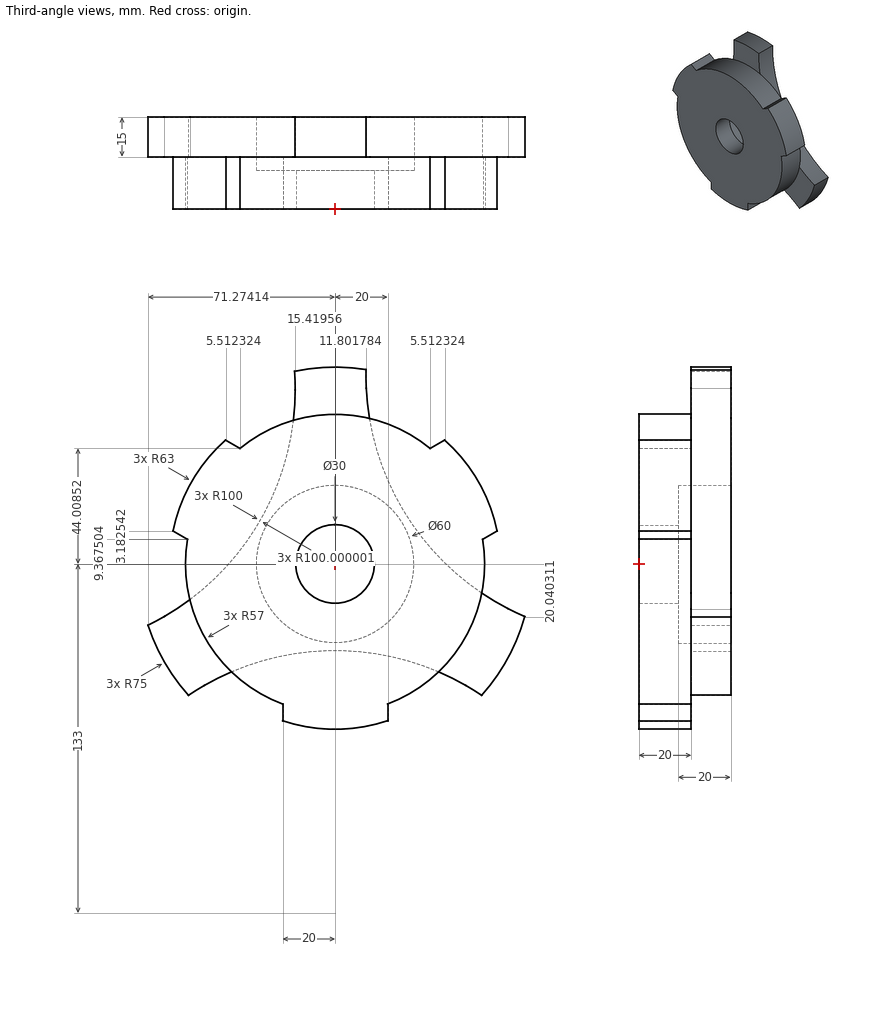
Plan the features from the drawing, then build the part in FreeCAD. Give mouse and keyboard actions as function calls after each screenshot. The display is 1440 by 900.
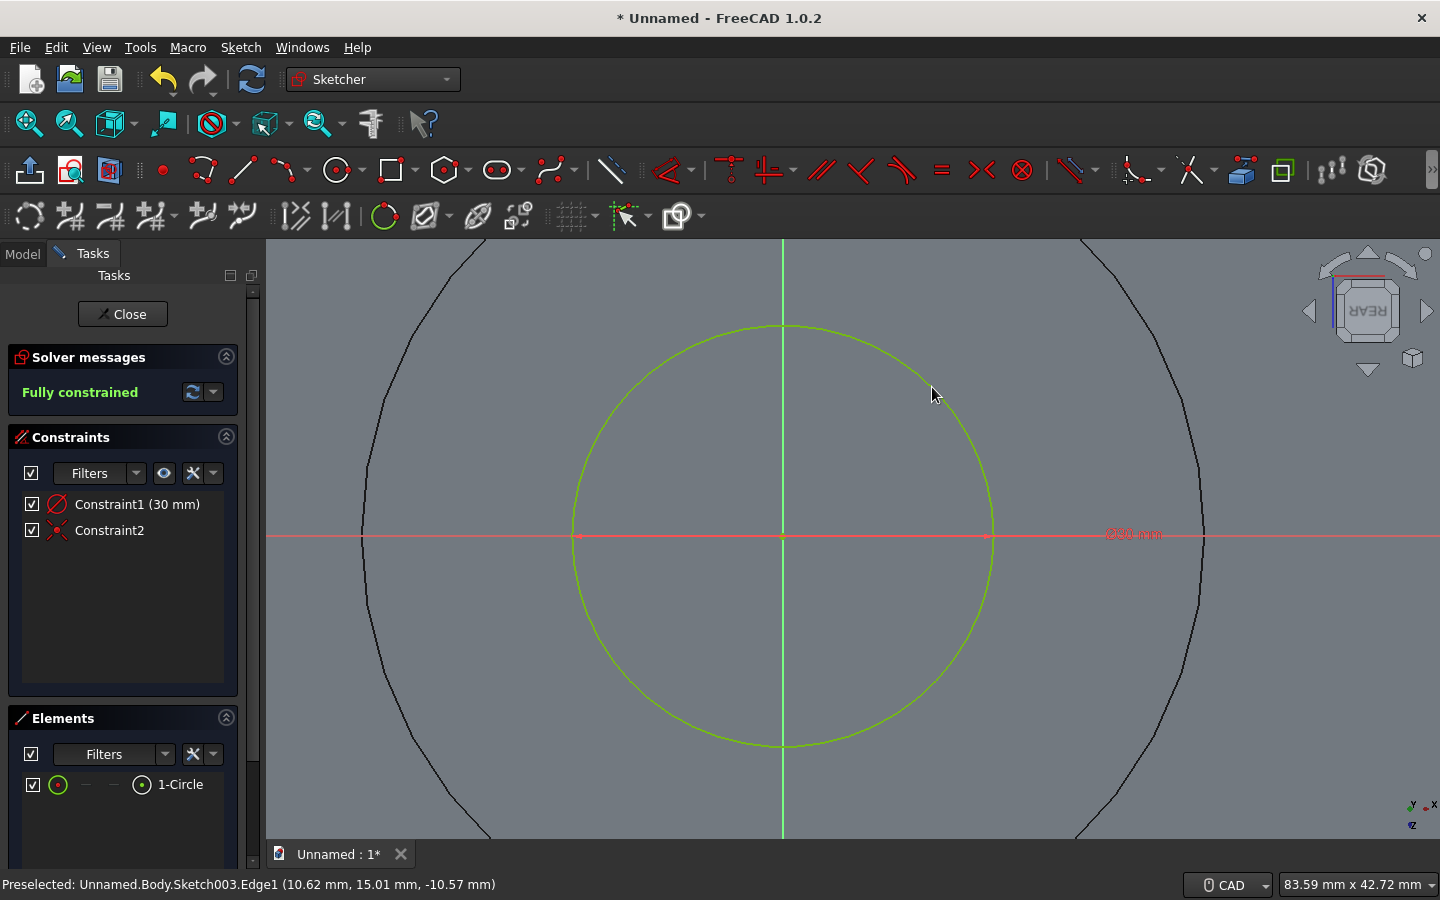
click(123, 314)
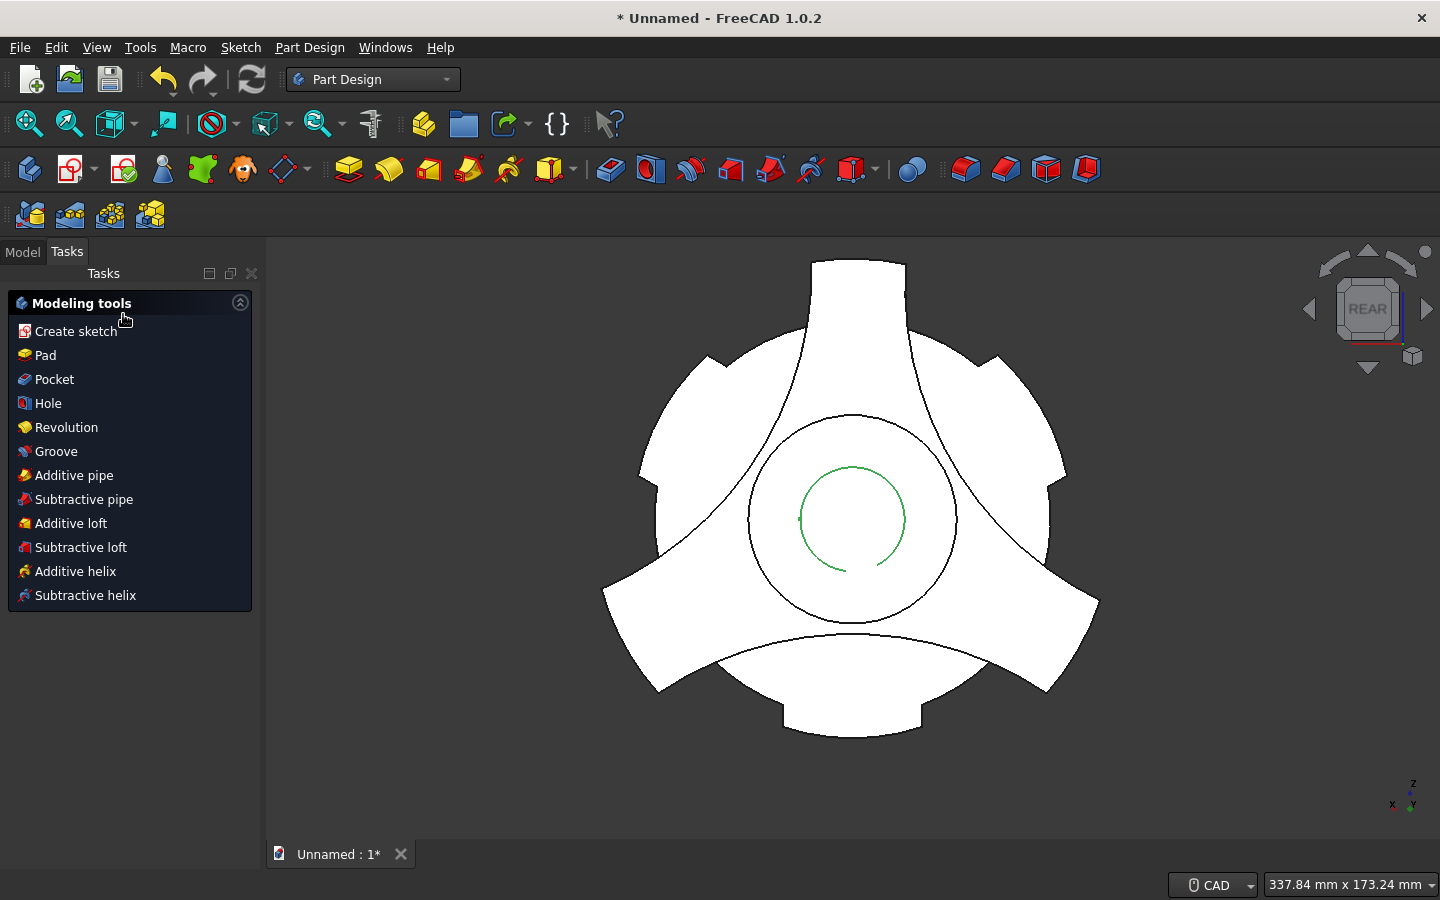
click(612, 170)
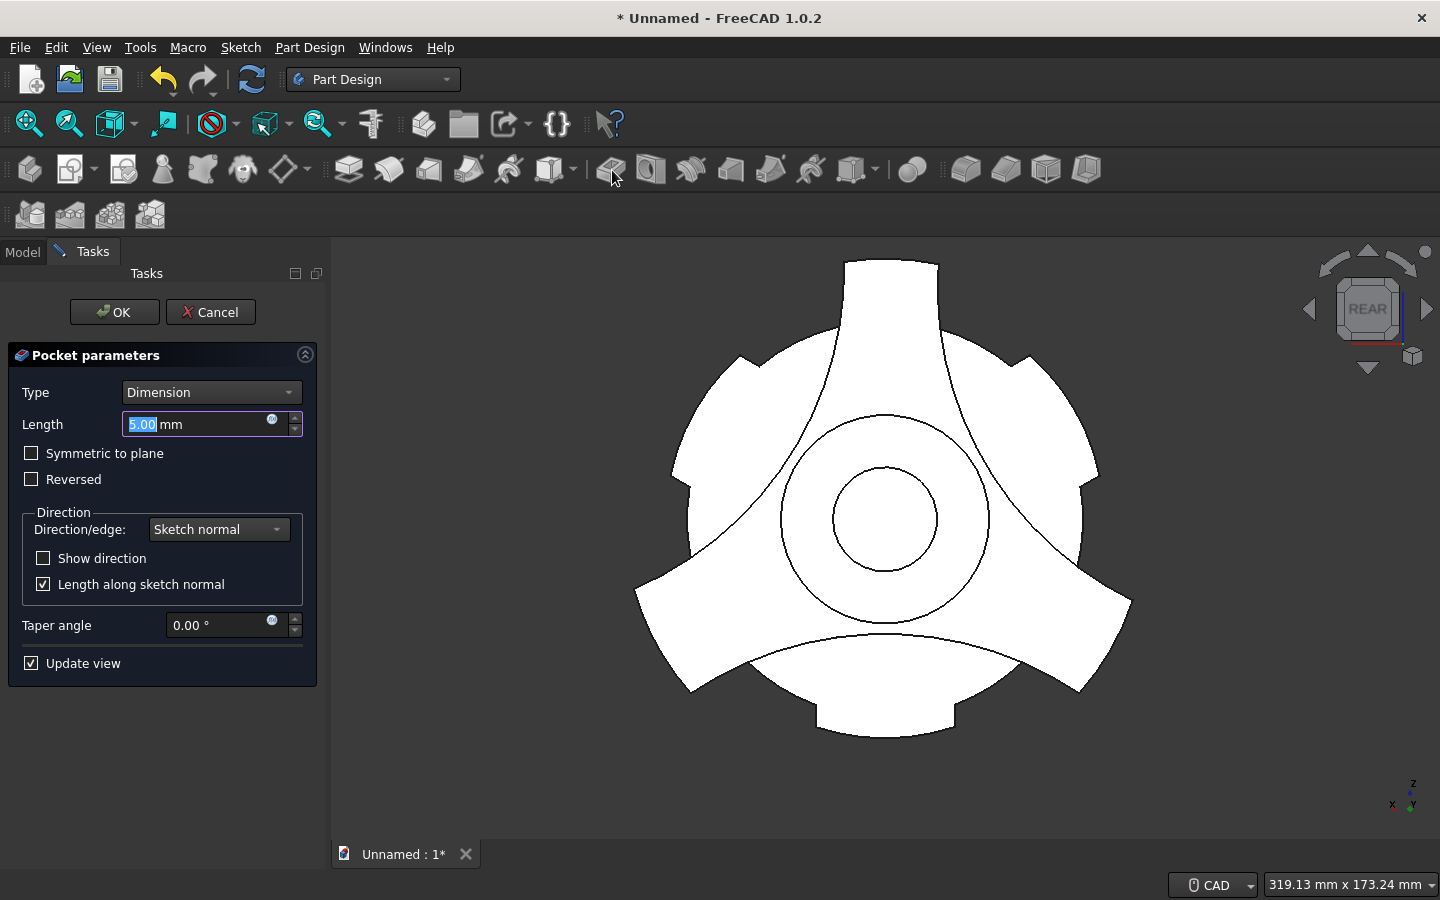
click(212, 392)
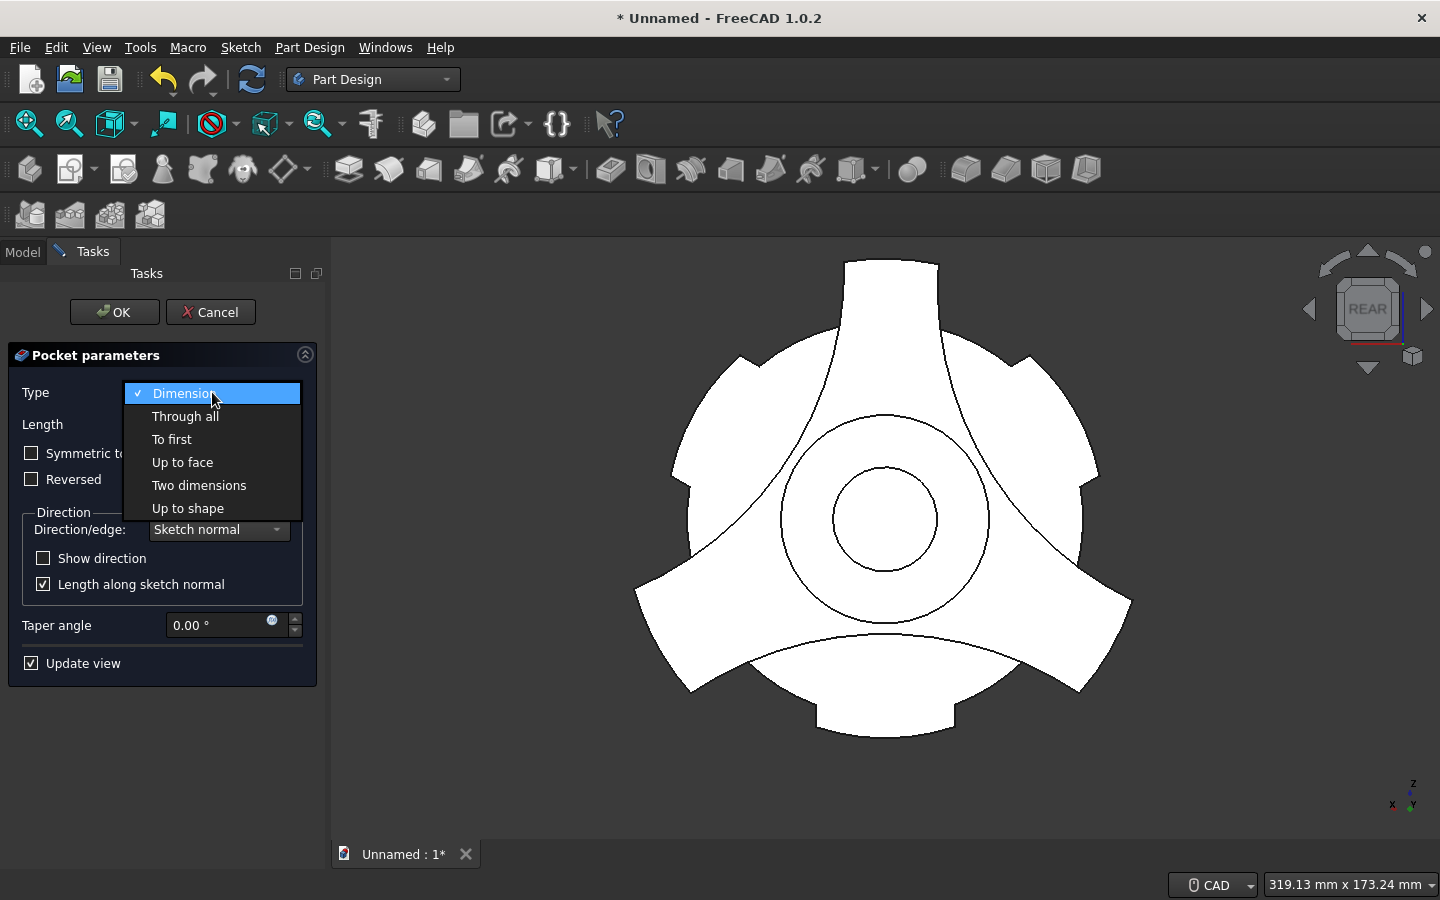
click(212, 416)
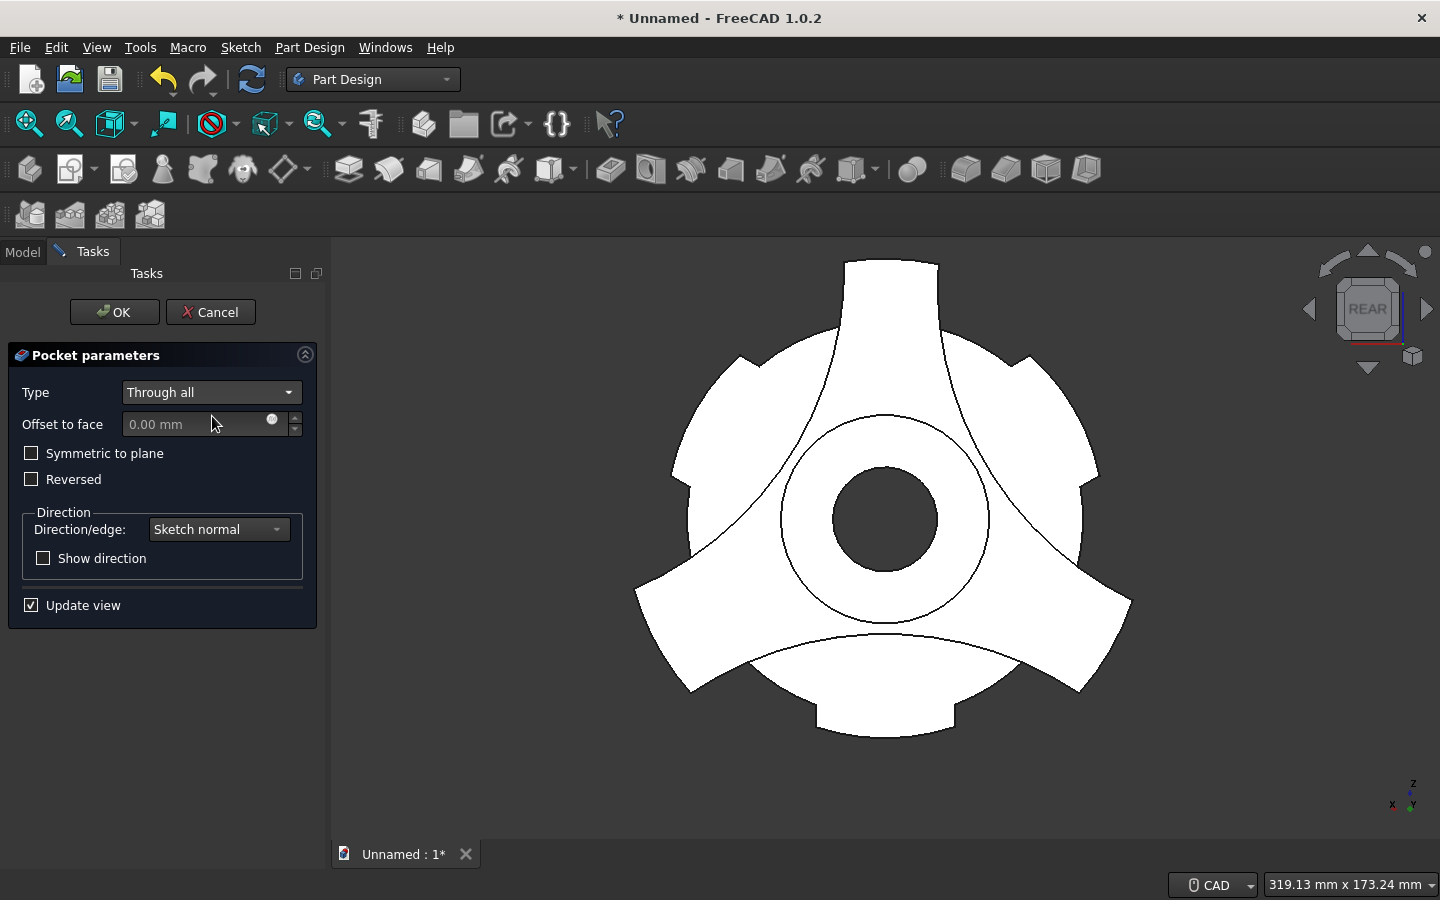
click(115, 312)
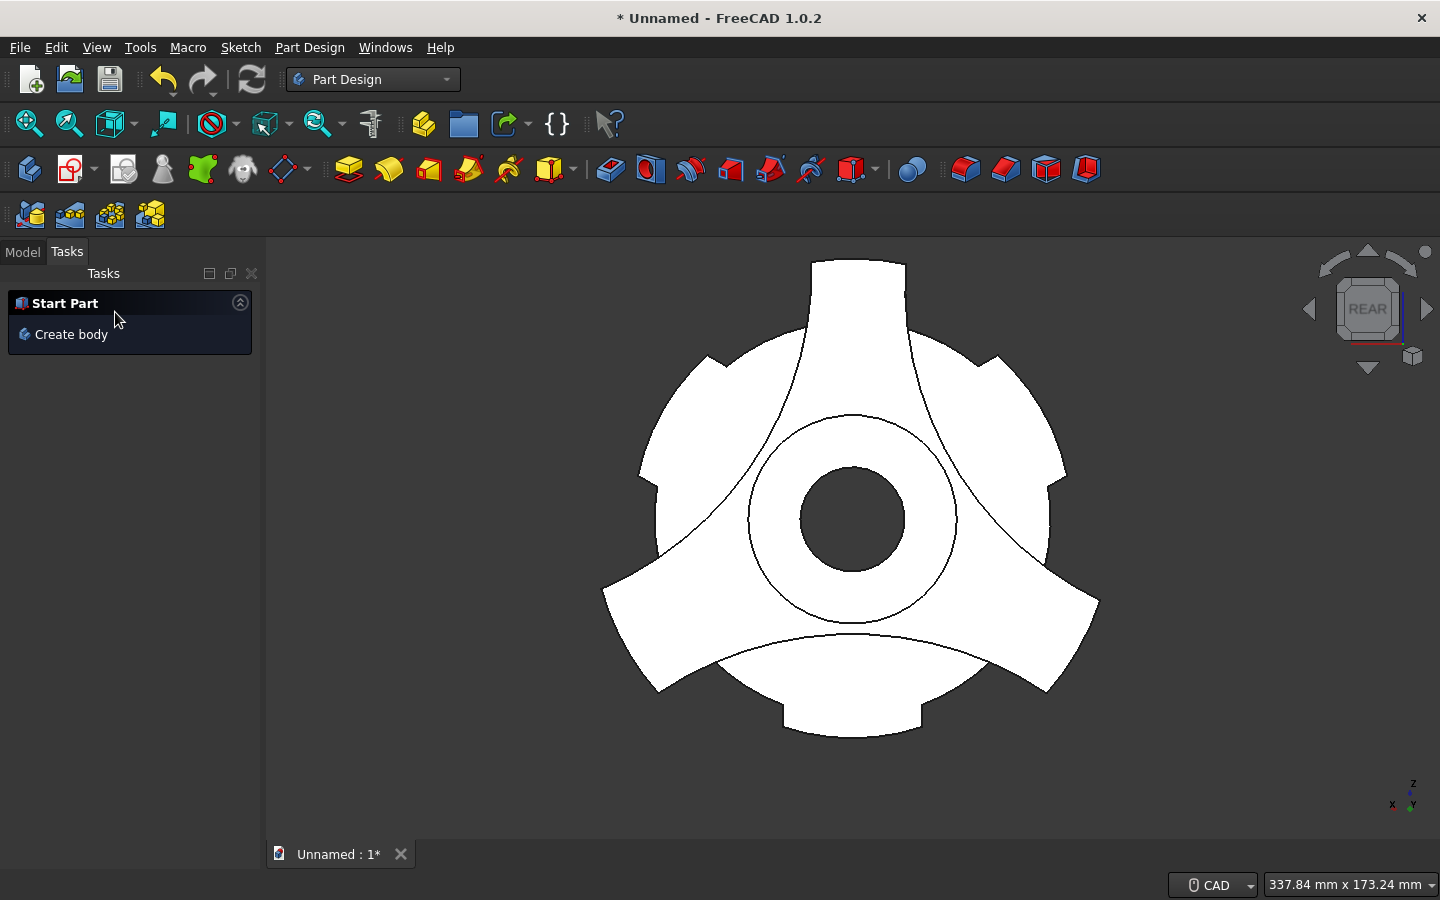
key(0)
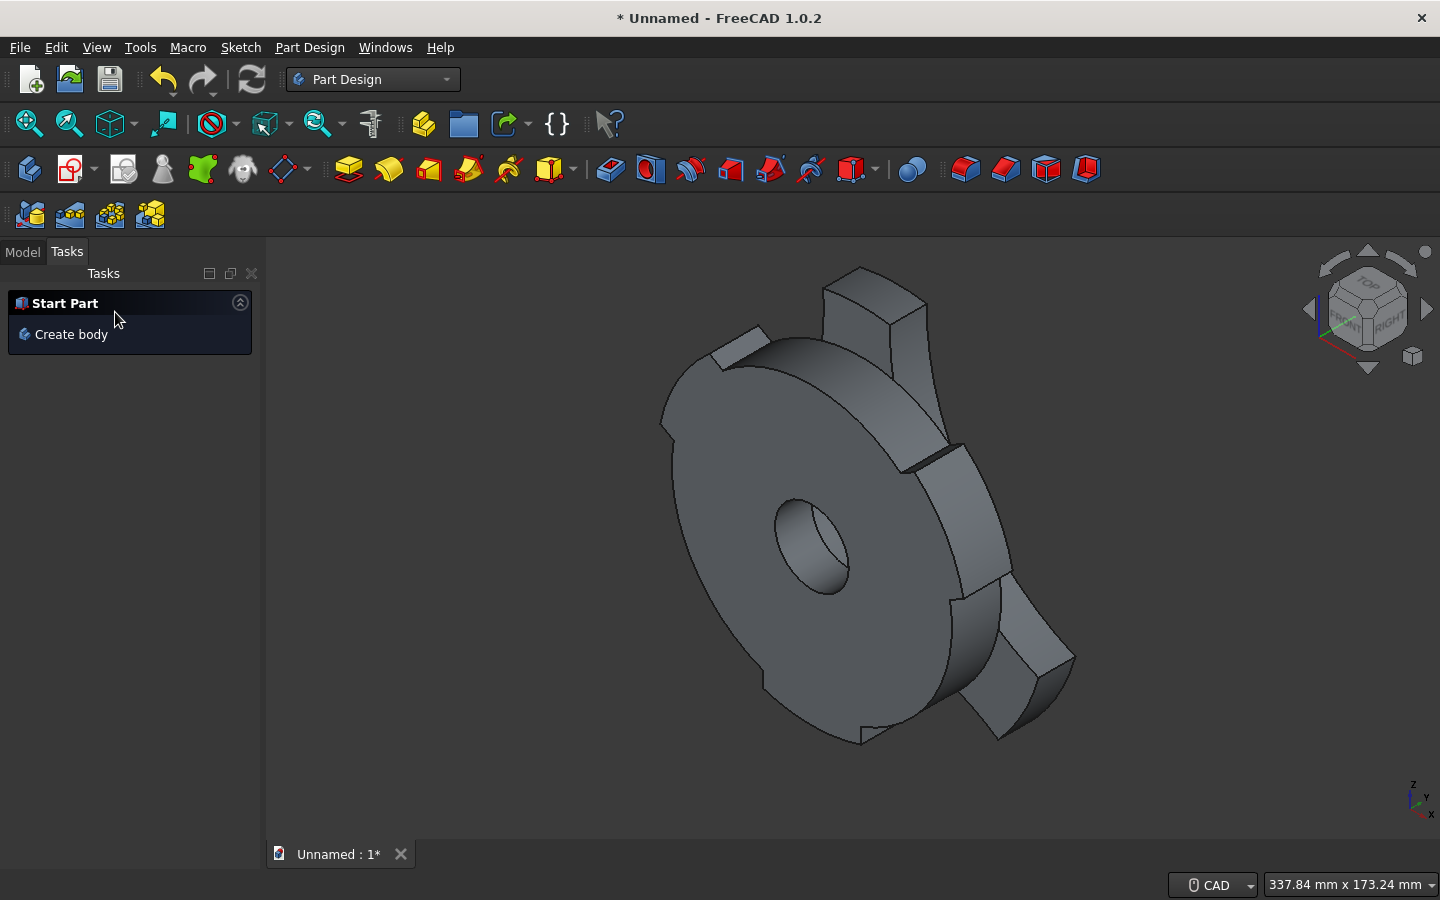
click(30, 124)